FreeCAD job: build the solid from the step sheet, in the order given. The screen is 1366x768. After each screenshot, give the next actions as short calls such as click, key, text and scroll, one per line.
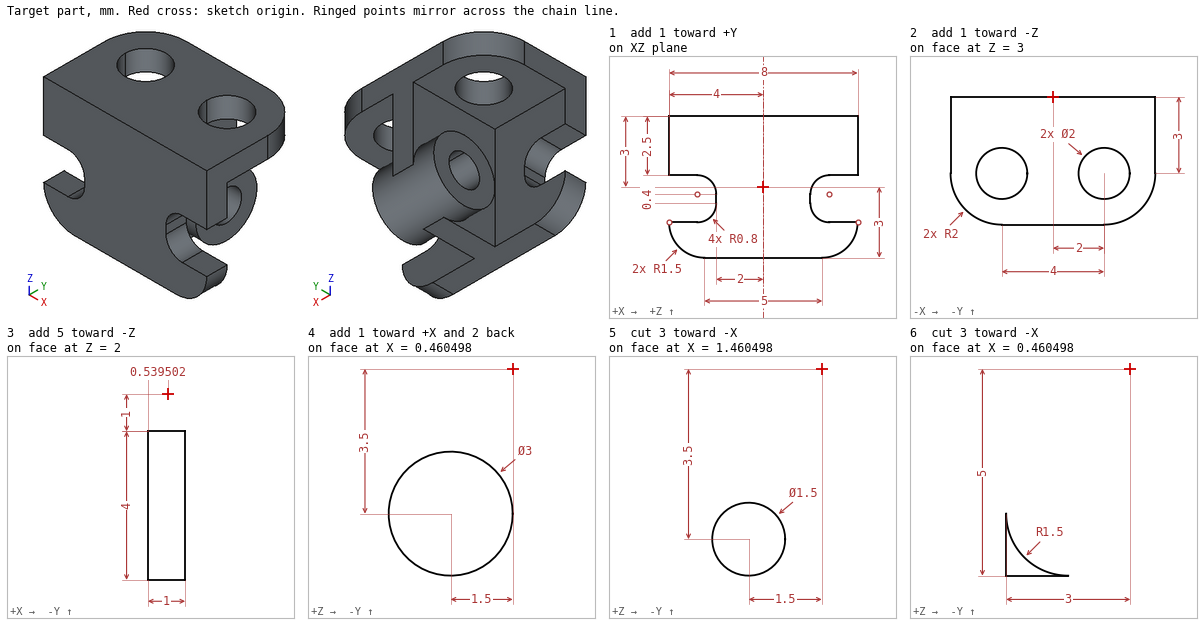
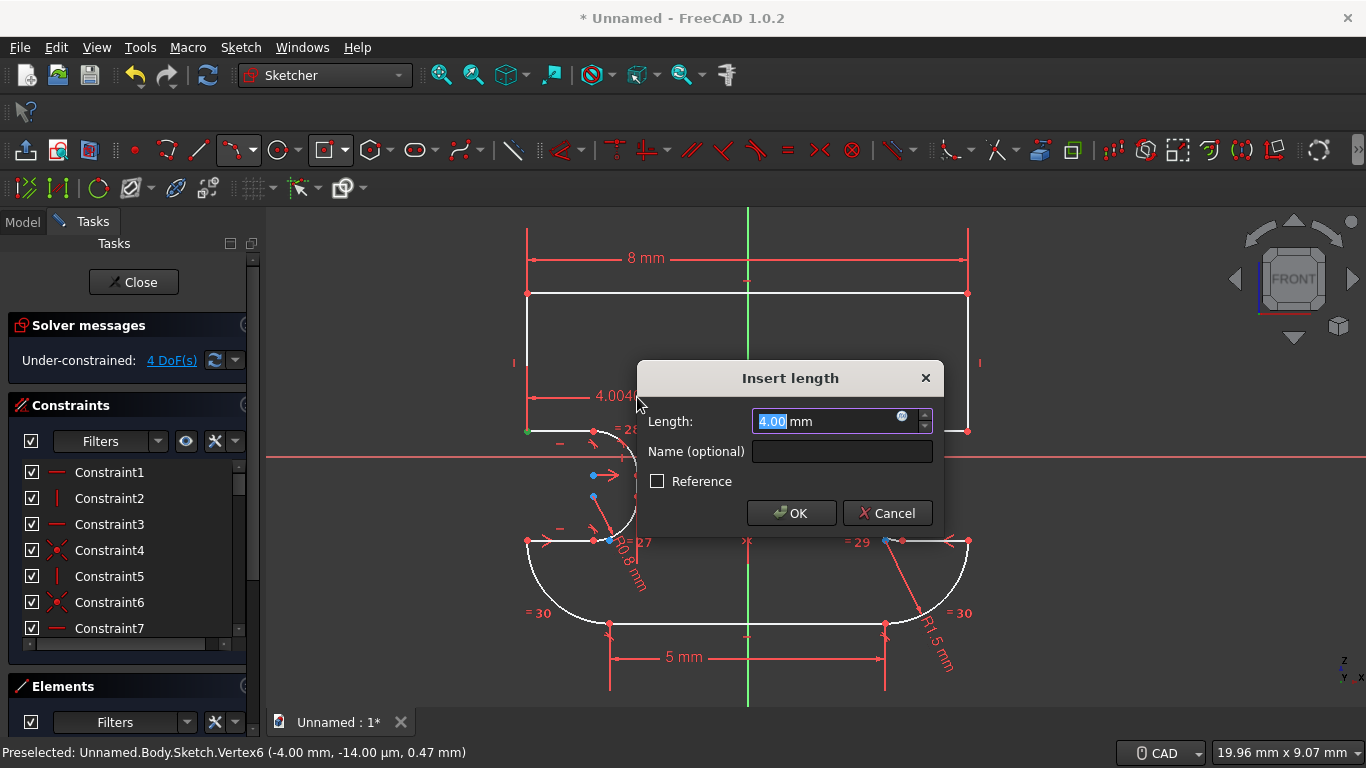
text(4)
key(Return)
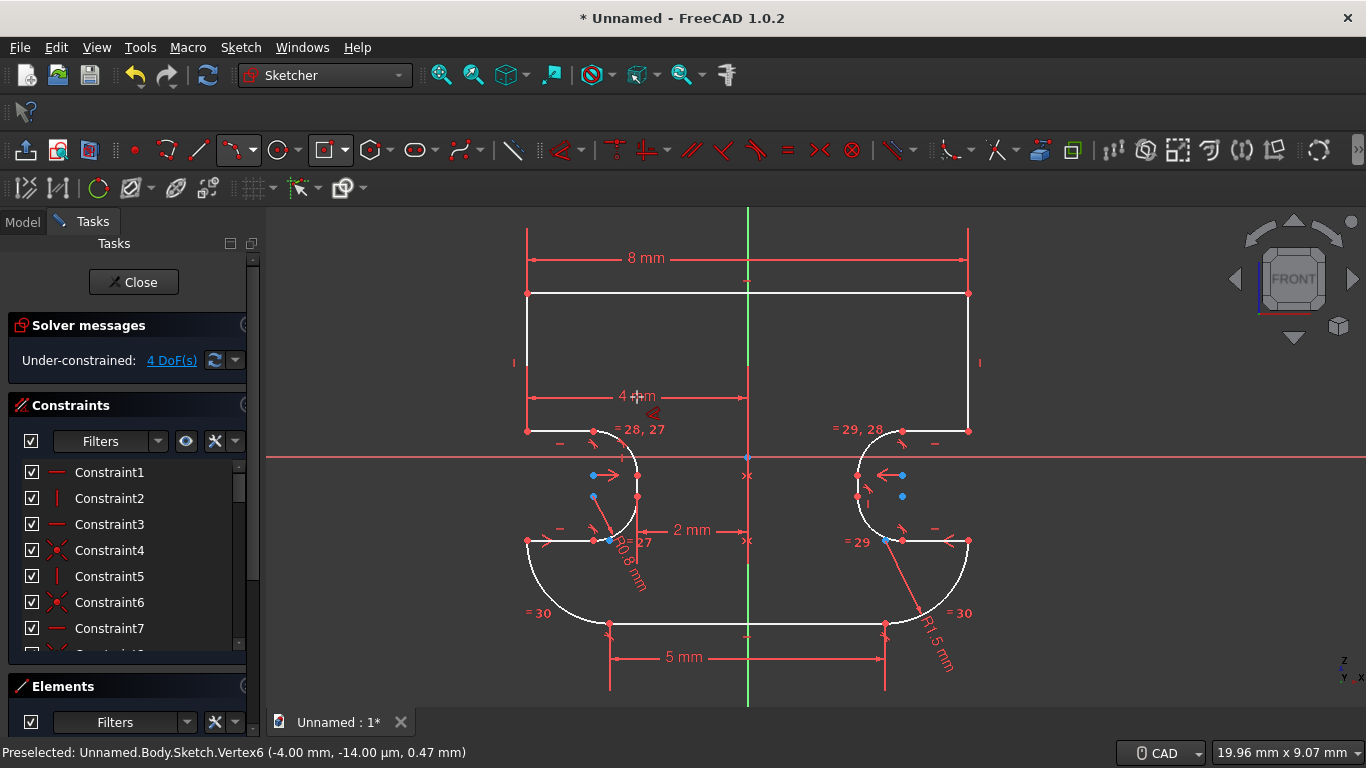
click(527, 293)
click(493, 375)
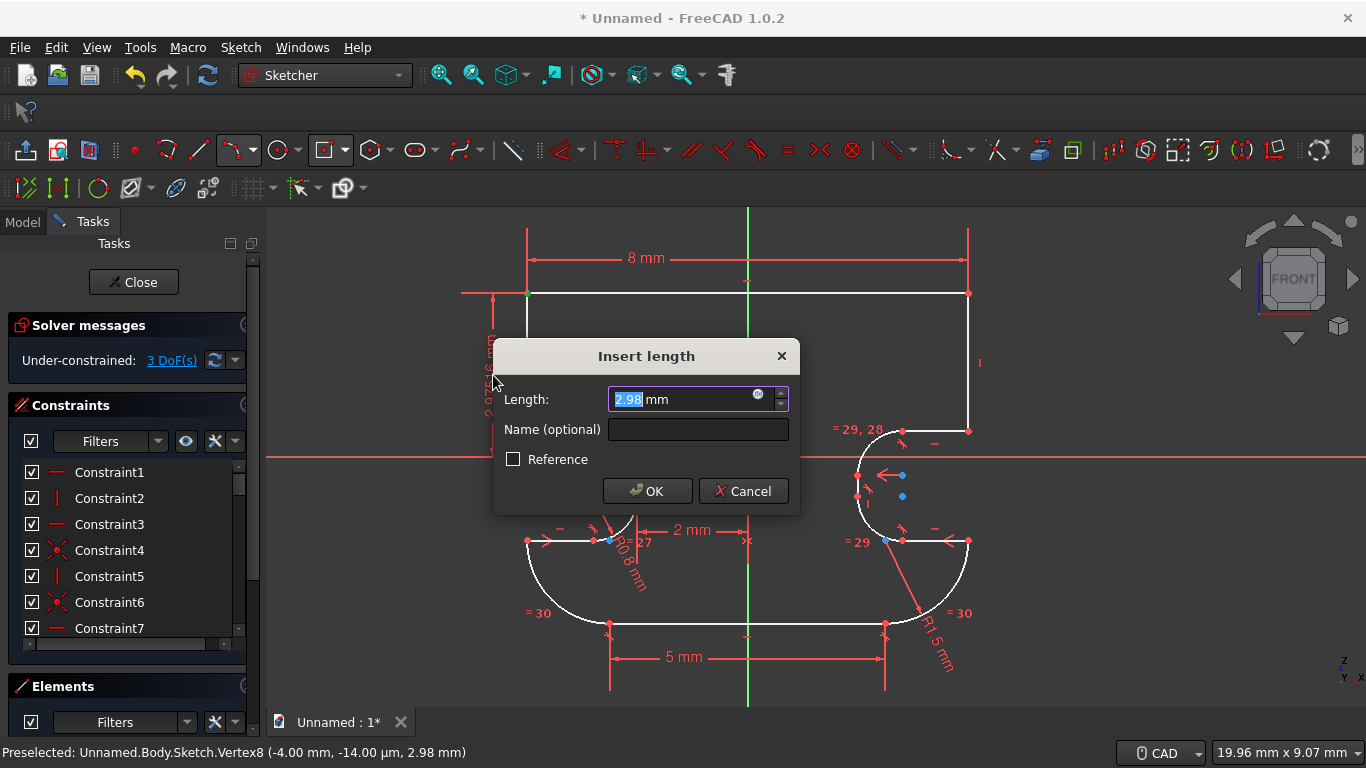
text(3)
key(Return)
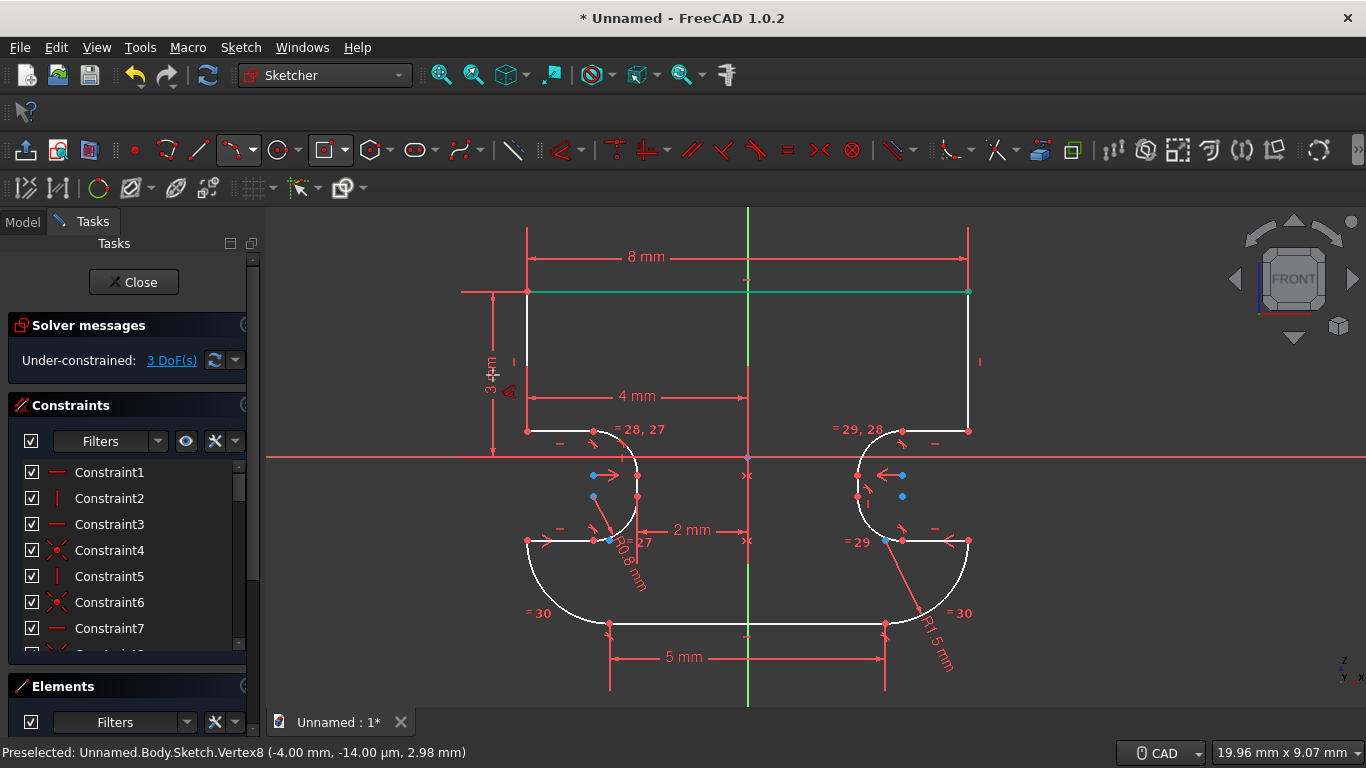
click(885, 624)
click(919, 502)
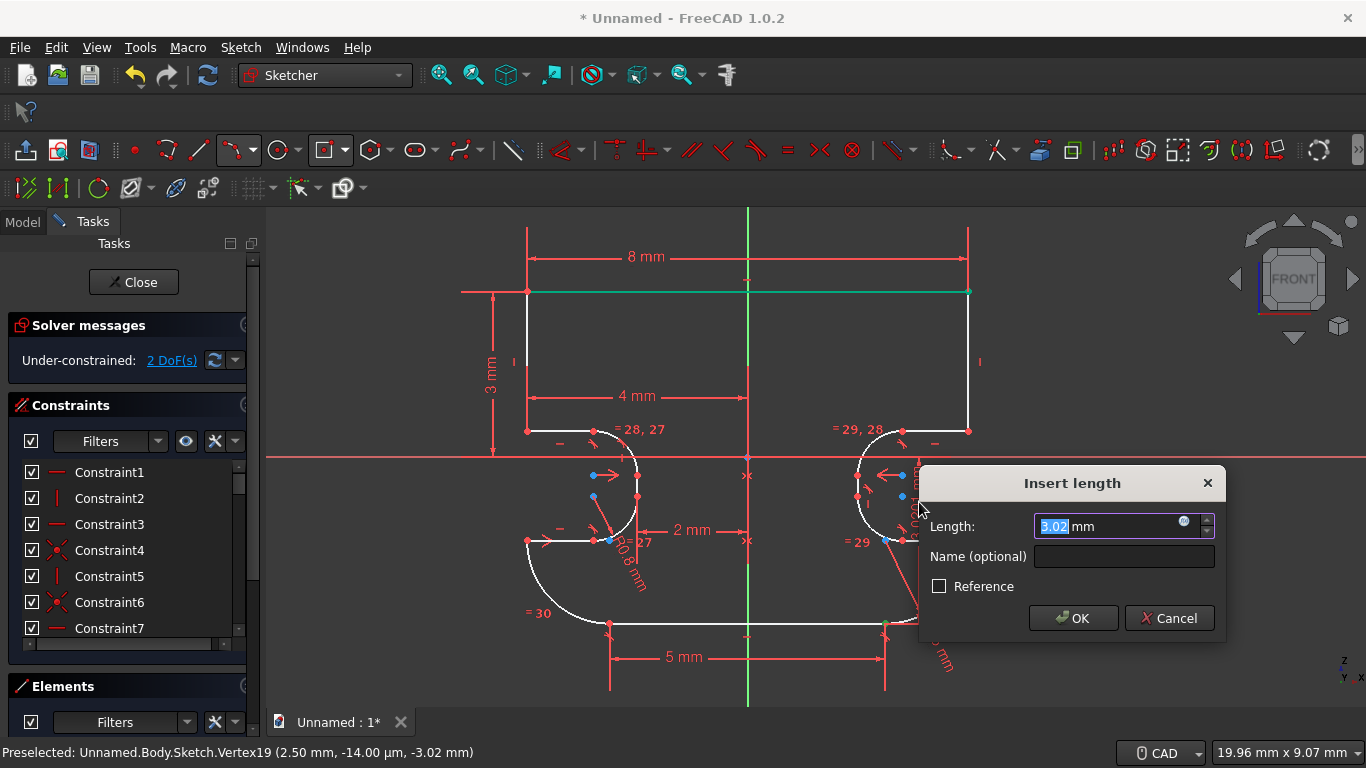
text(3)
key(Return)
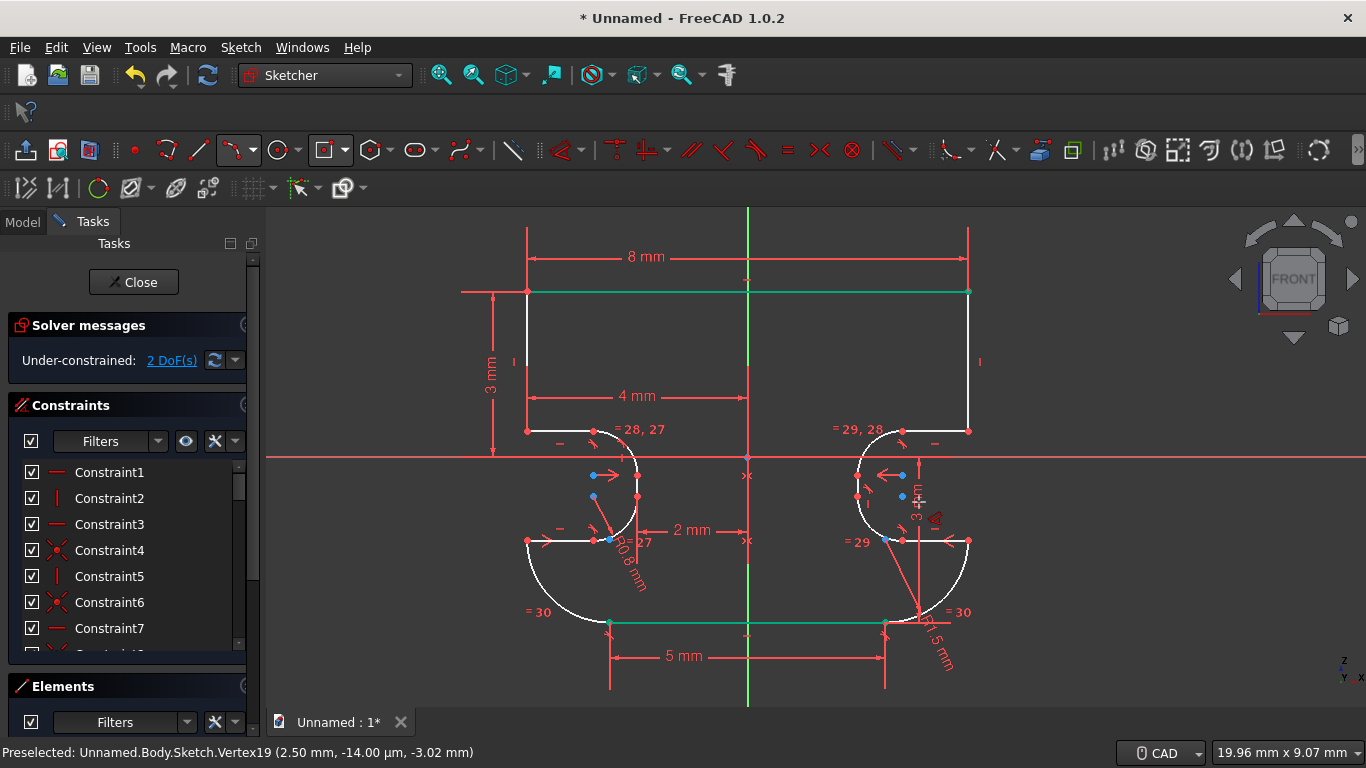
scroll(637, 486, up, 3)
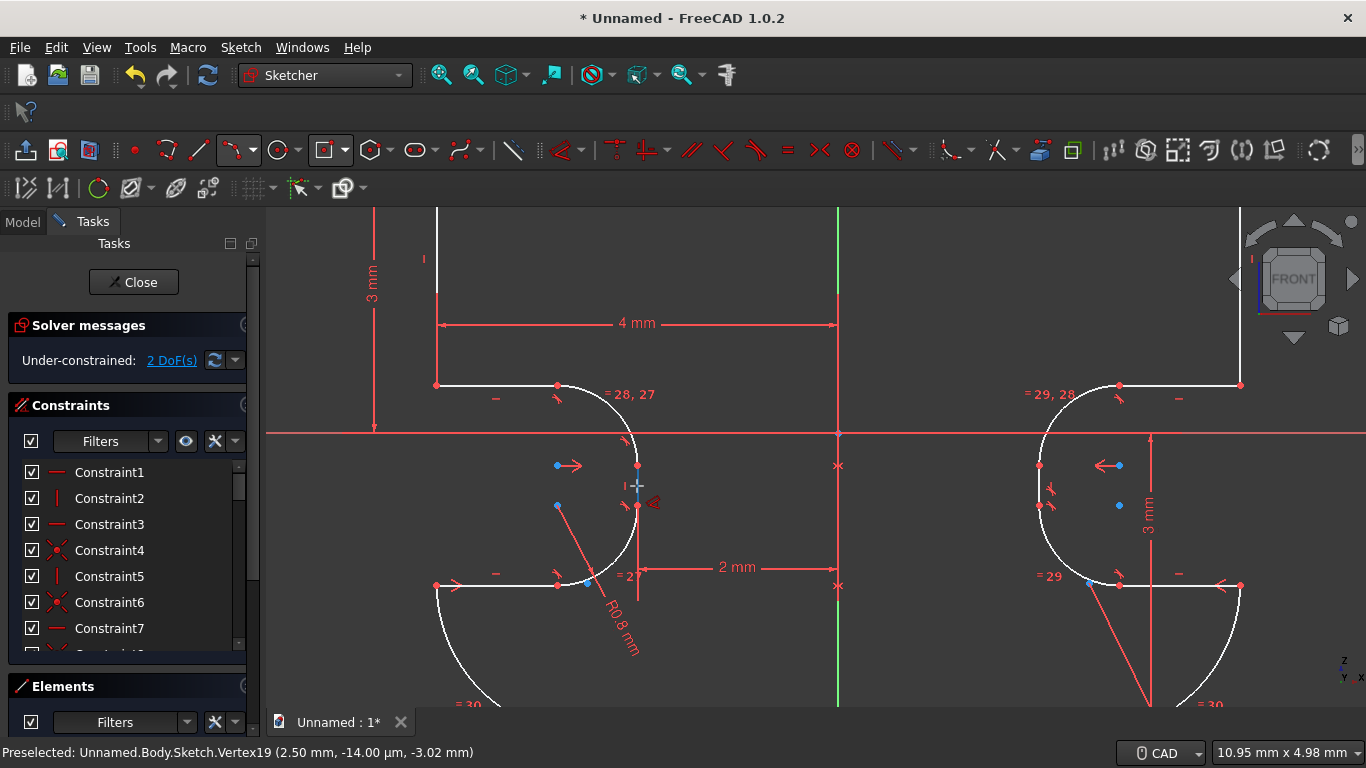
click(638, 486)
click(604, 486)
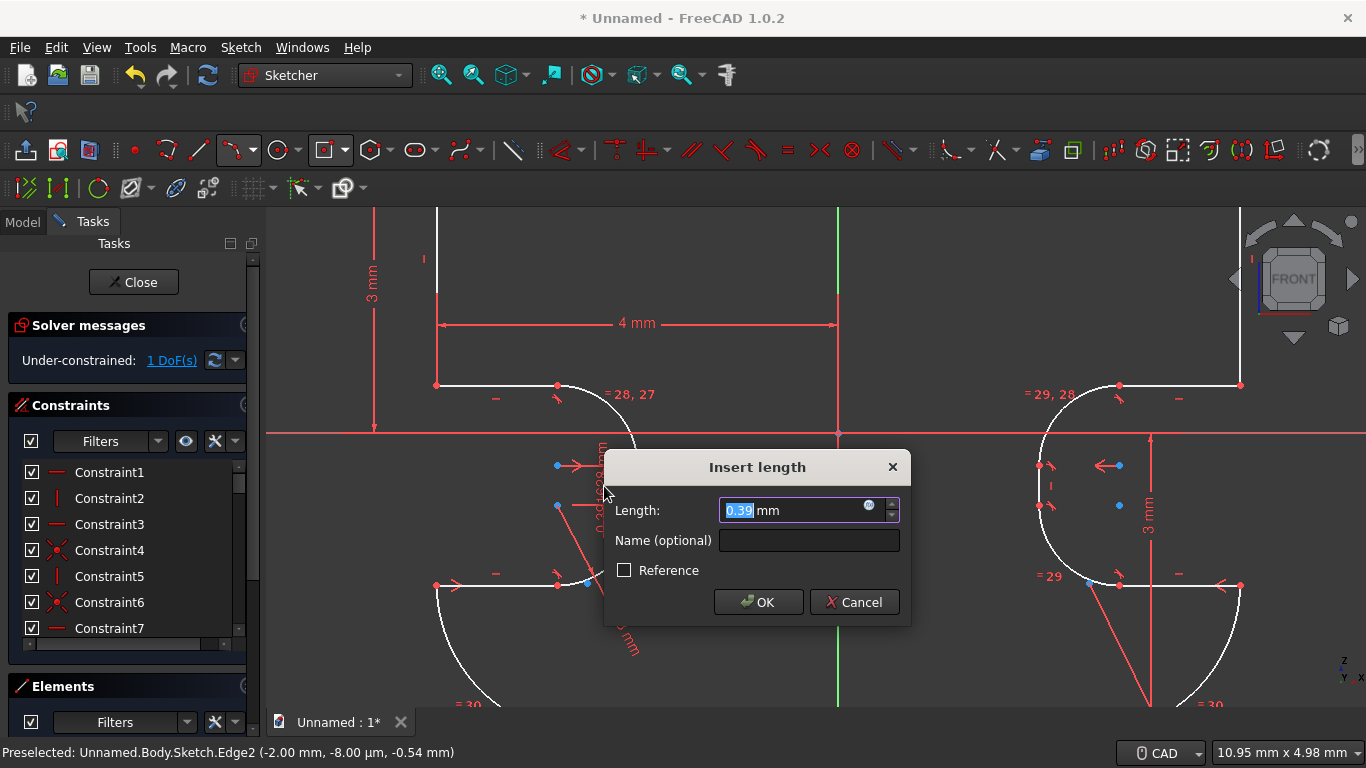
text(0.4)
key(Return)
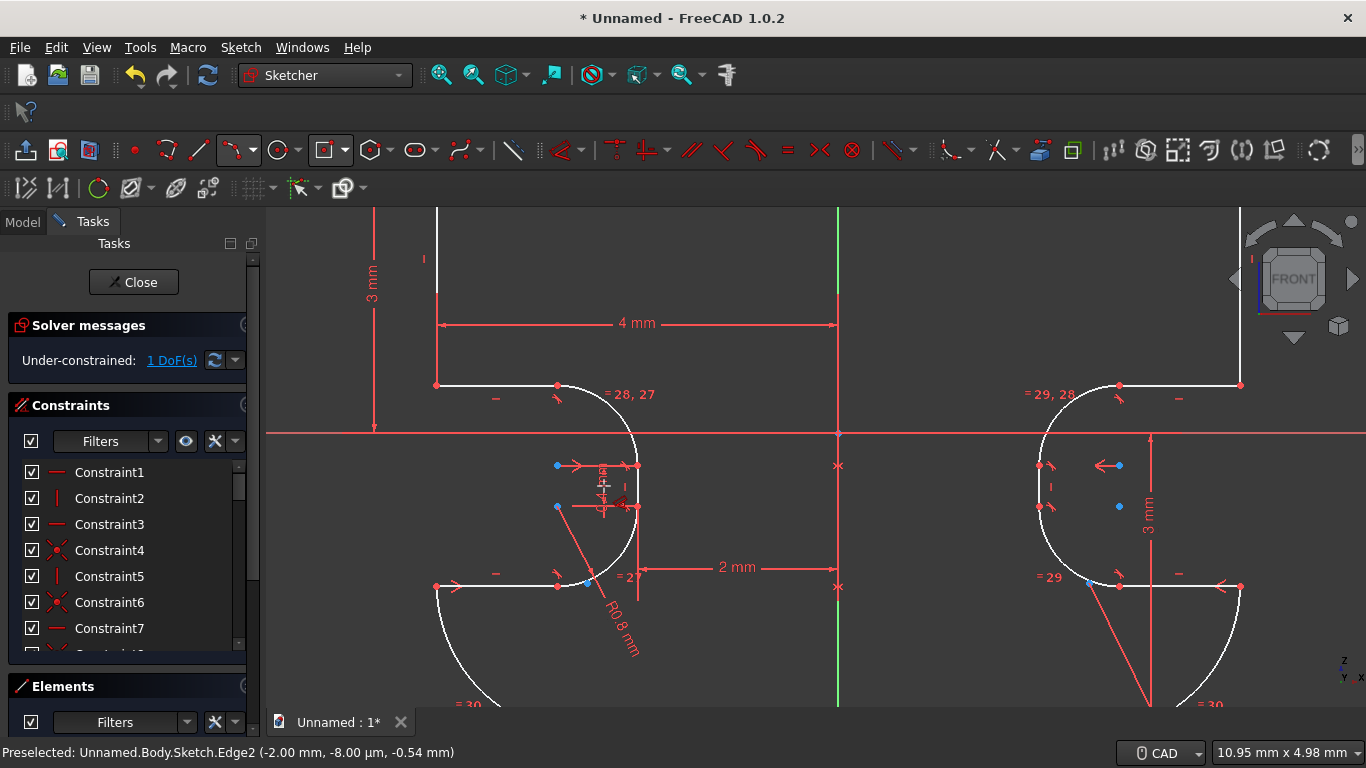
click(437, 309)
click(403, 310)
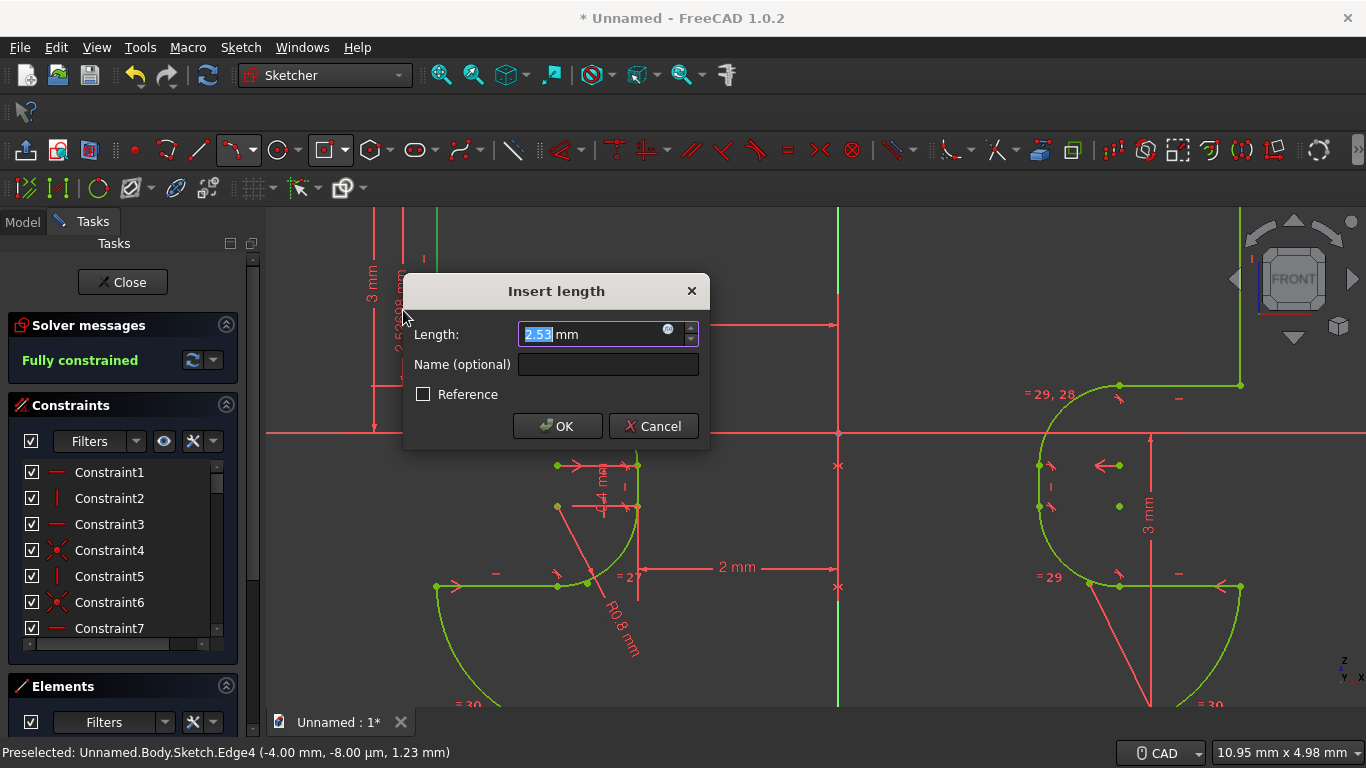
text(2.5)
key(Return)
key(Escape)